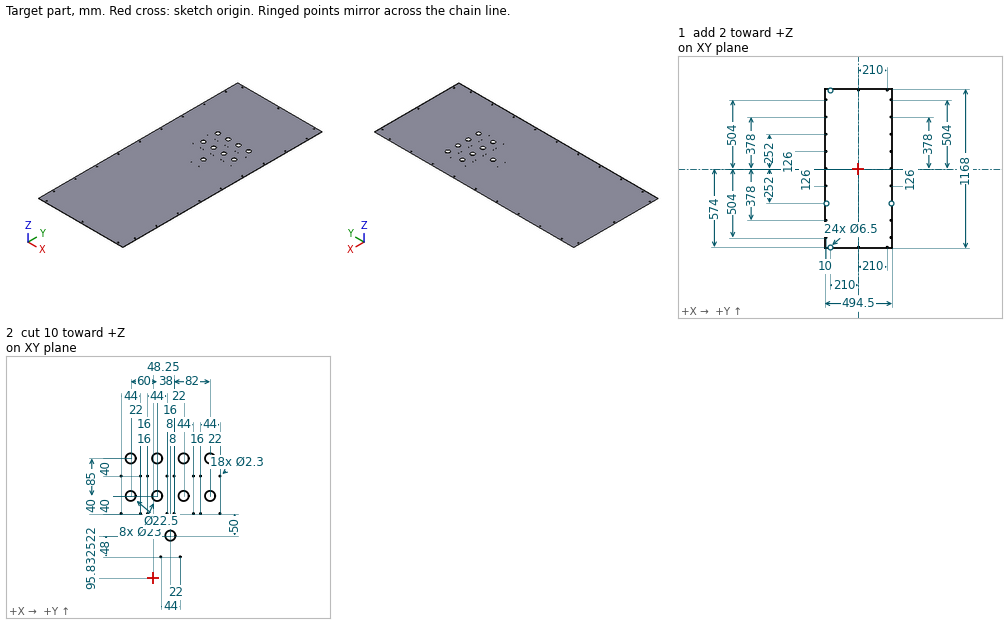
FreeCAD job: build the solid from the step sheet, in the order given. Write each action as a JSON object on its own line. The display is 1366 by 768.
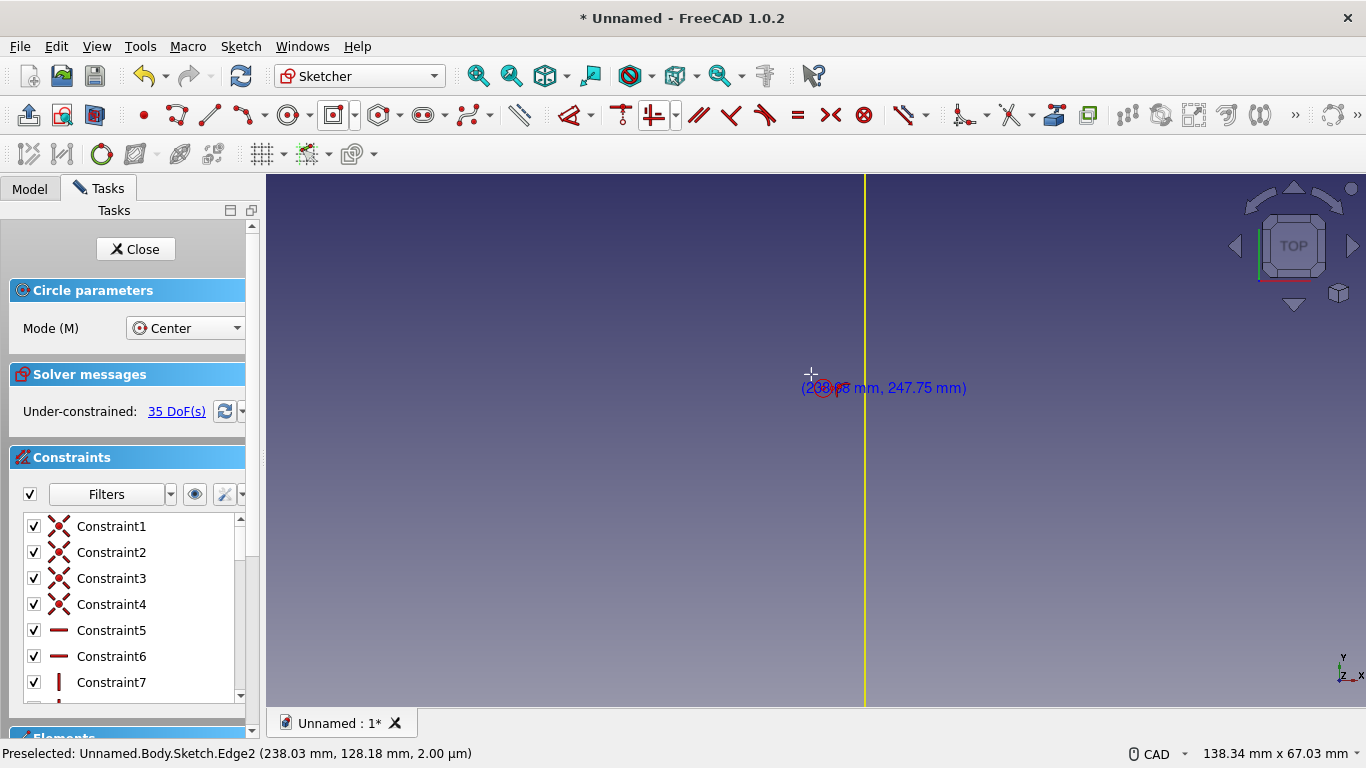
{"action": "scroll", "coordinate": [826, 359], "scroll_direction": "down", "scroll_amount": 16}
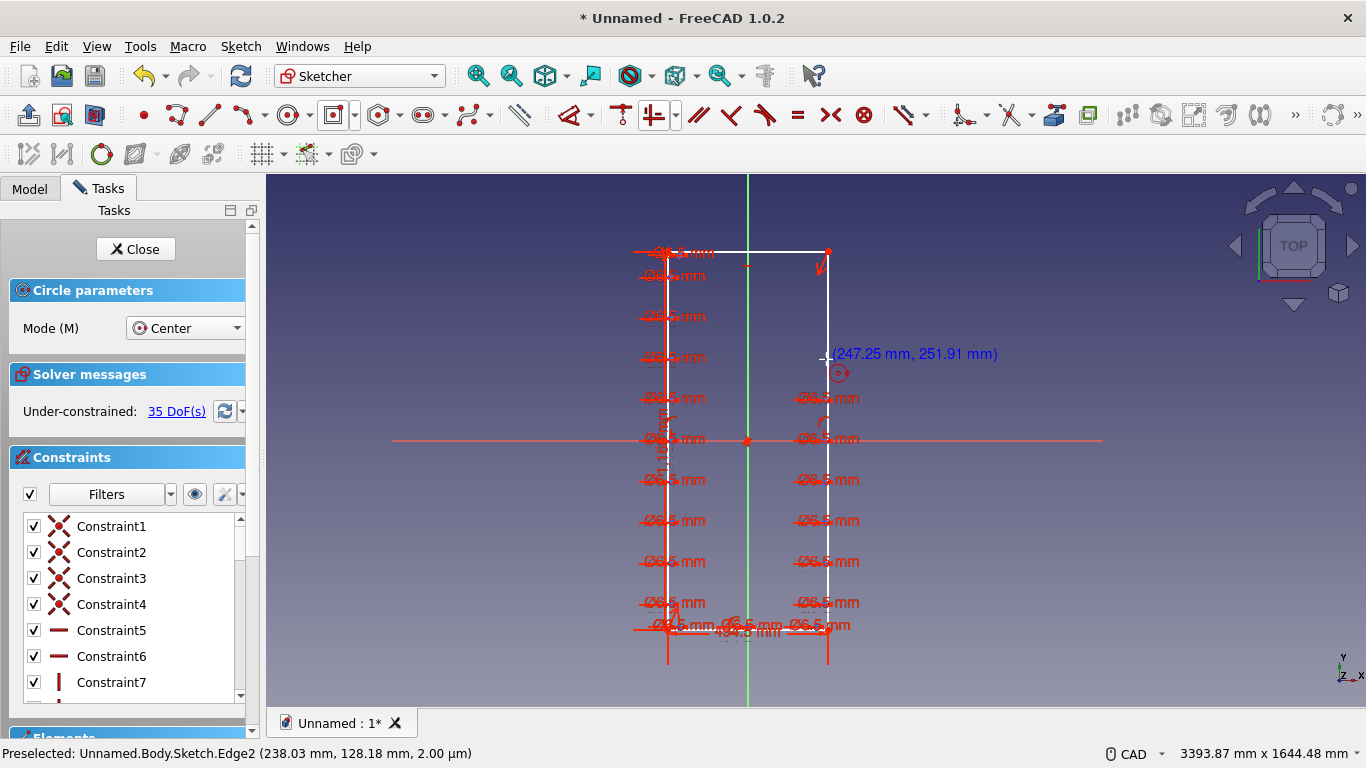
{"action": "scroll", "coordinate": [825, 359], "scroll_direction": "up", "scroll_amount": 8}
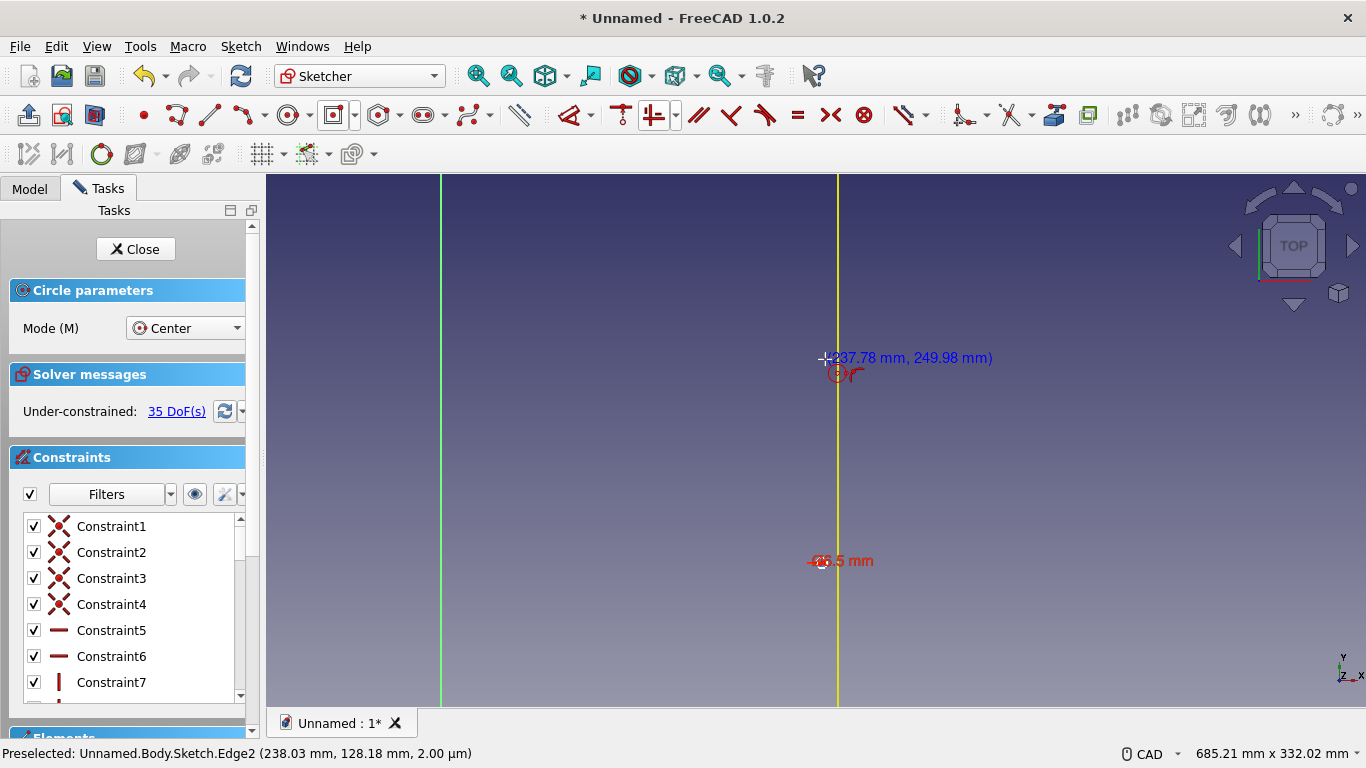
{"action": "left_click", "coordinate": [822, 359]}
{"action": "mouse_move", "coordinate": [818, 356]}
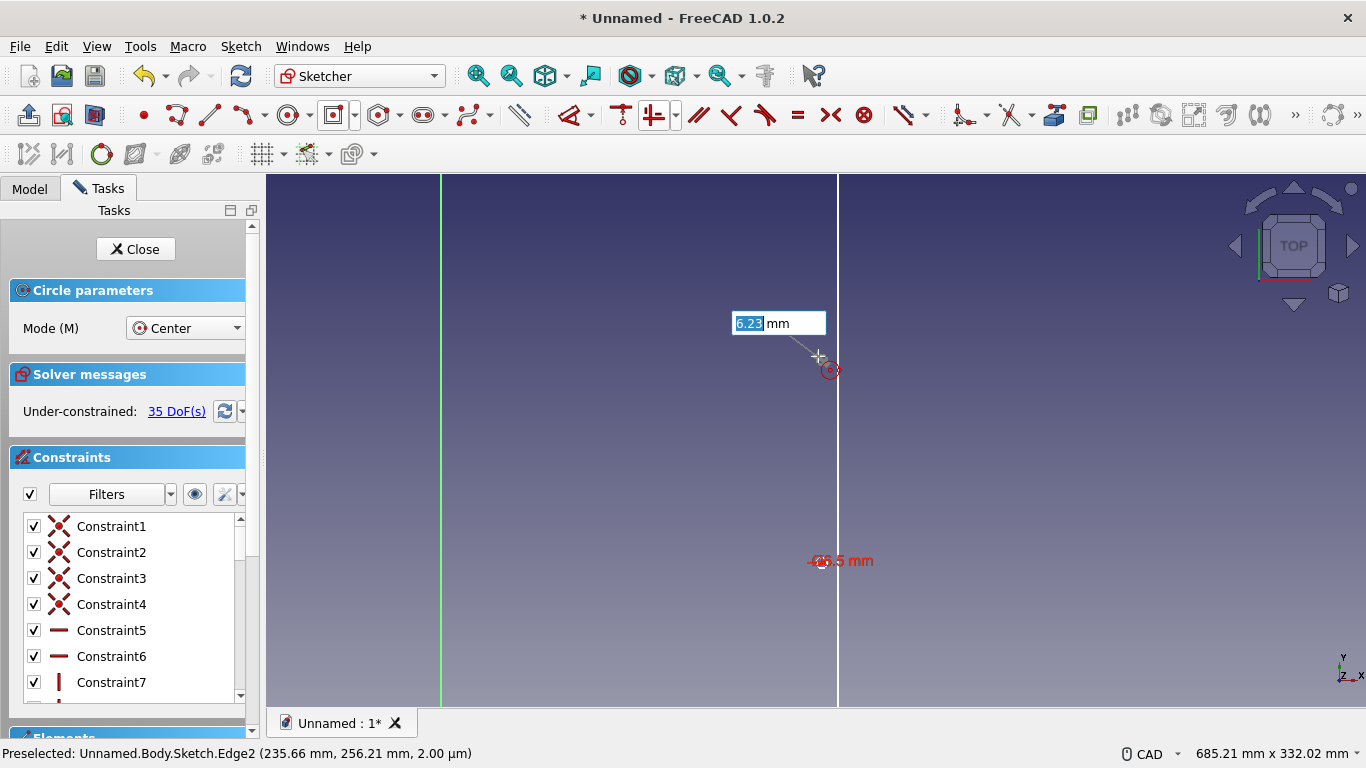
{"action": "type", "text": "6.5"}
{"action": "key", "text": "Return"}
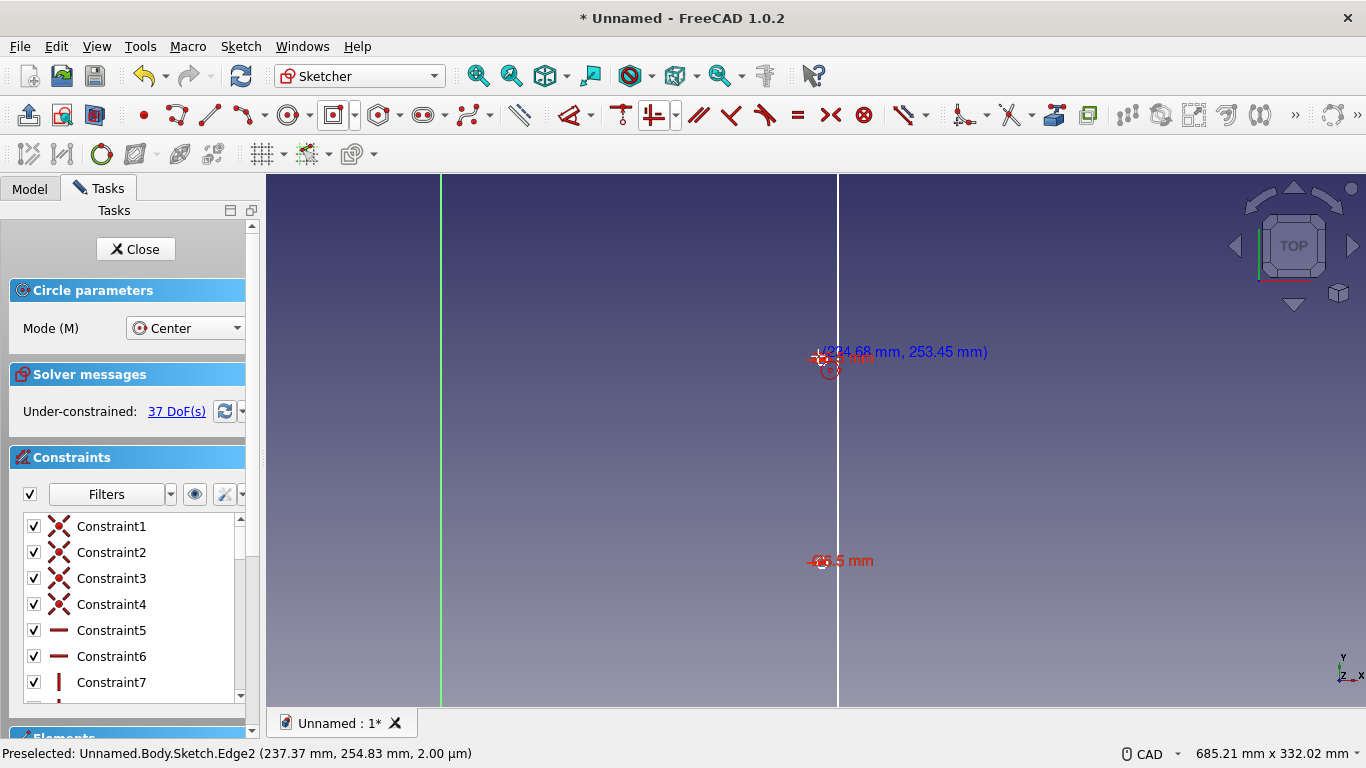
{"action": "scroll", "coordinate": [808, 376], "scroll_direction": "down", "scroll_amount": 9}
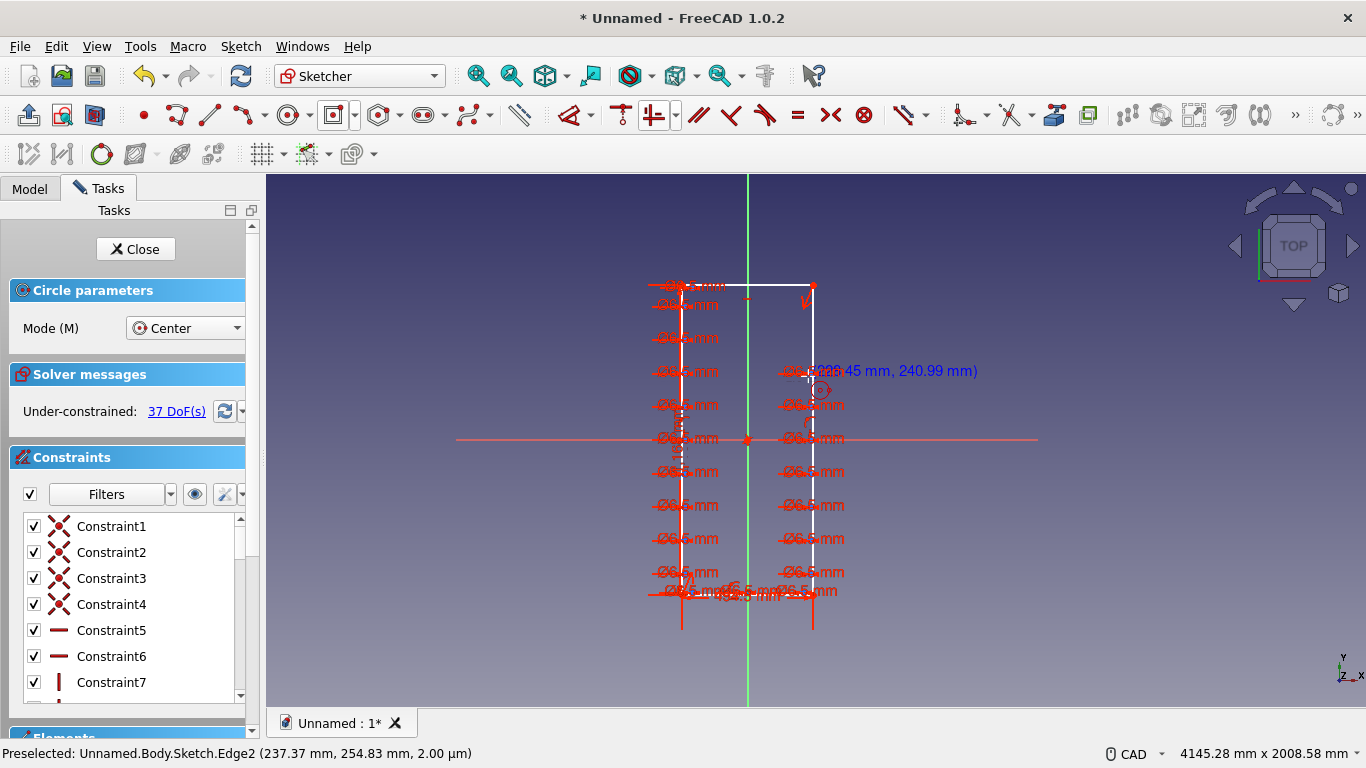
{"action": "scroll", "coordinate": [748, 288], "scroll_direction": "up", "scroll_amount": 17}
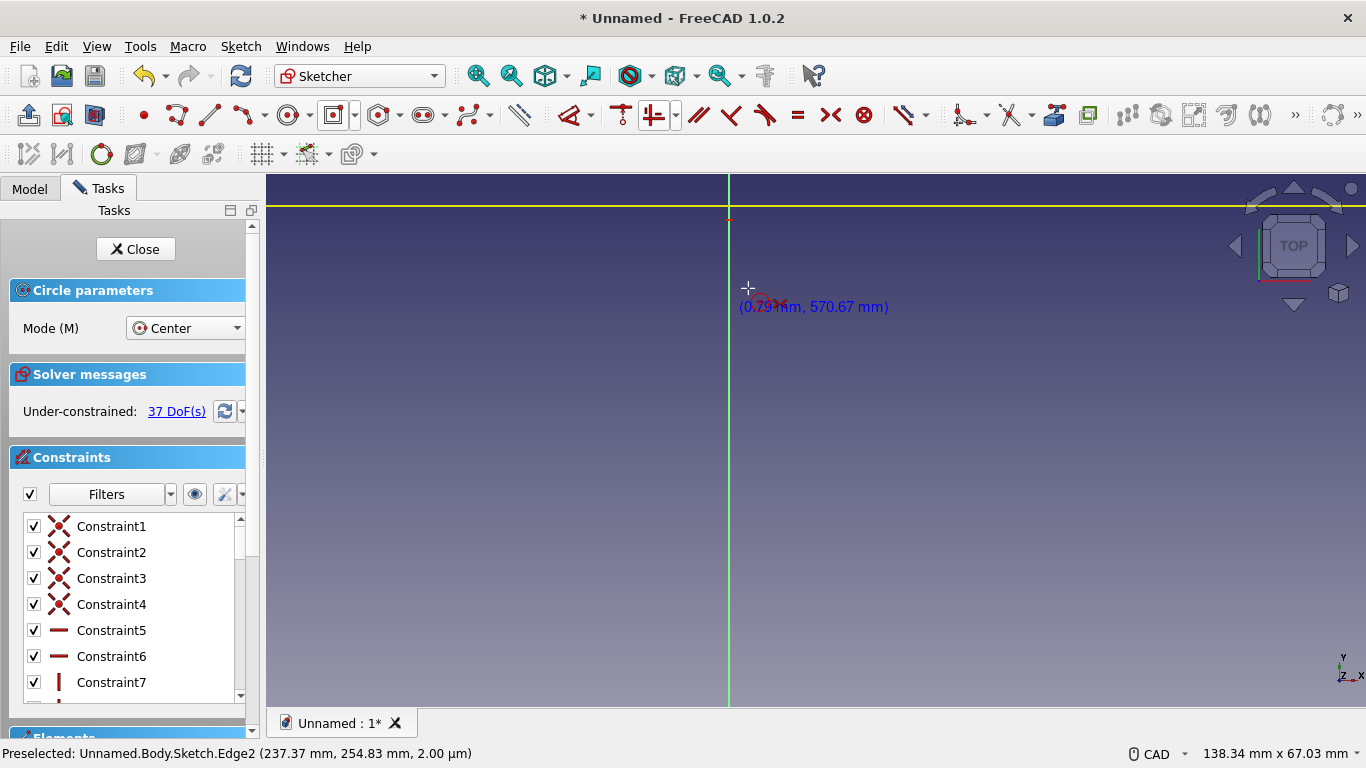
{"action": "scroll", "coordinate": [748, 253], "scroll_direction": "down", "scroll_amount": 16}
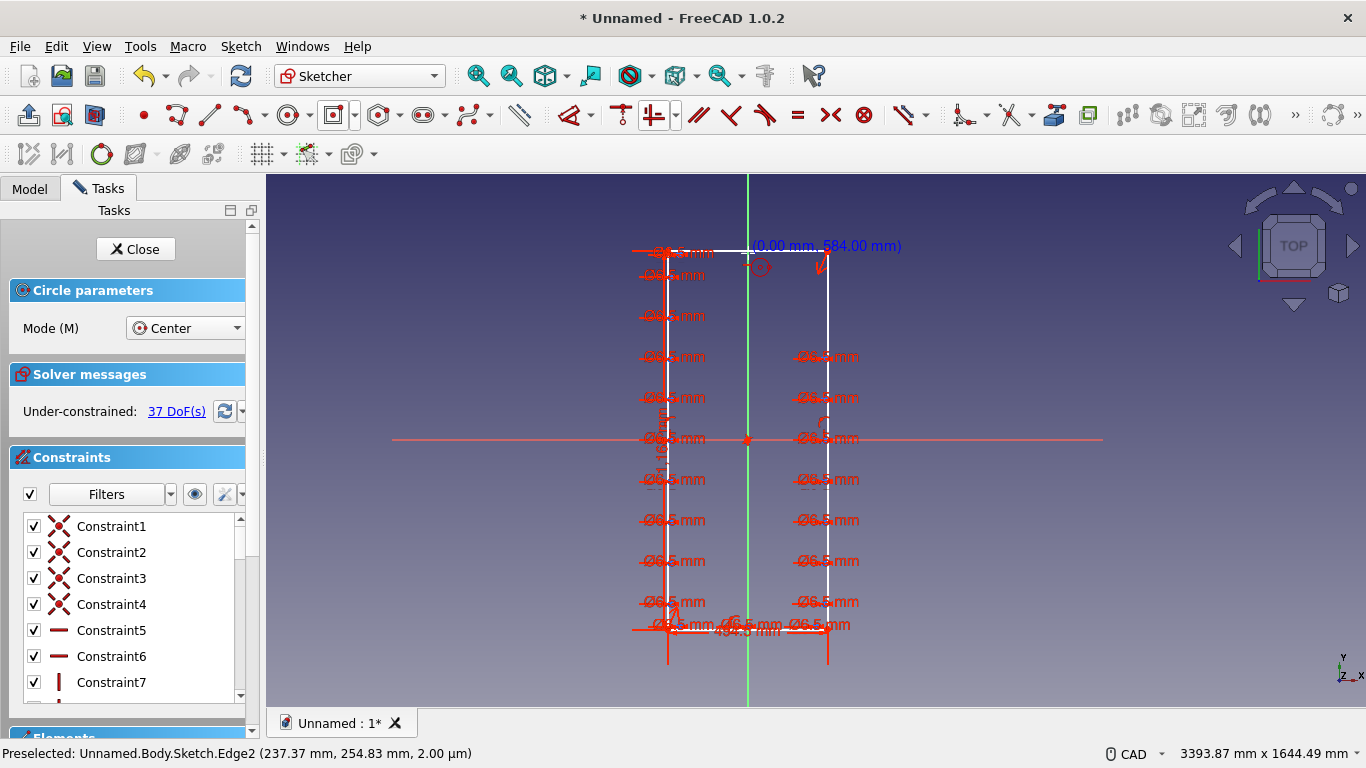
{"action": "scroll", "coordinate": [748, 254], "scroll_direction": "up", "scroll_amount": 8}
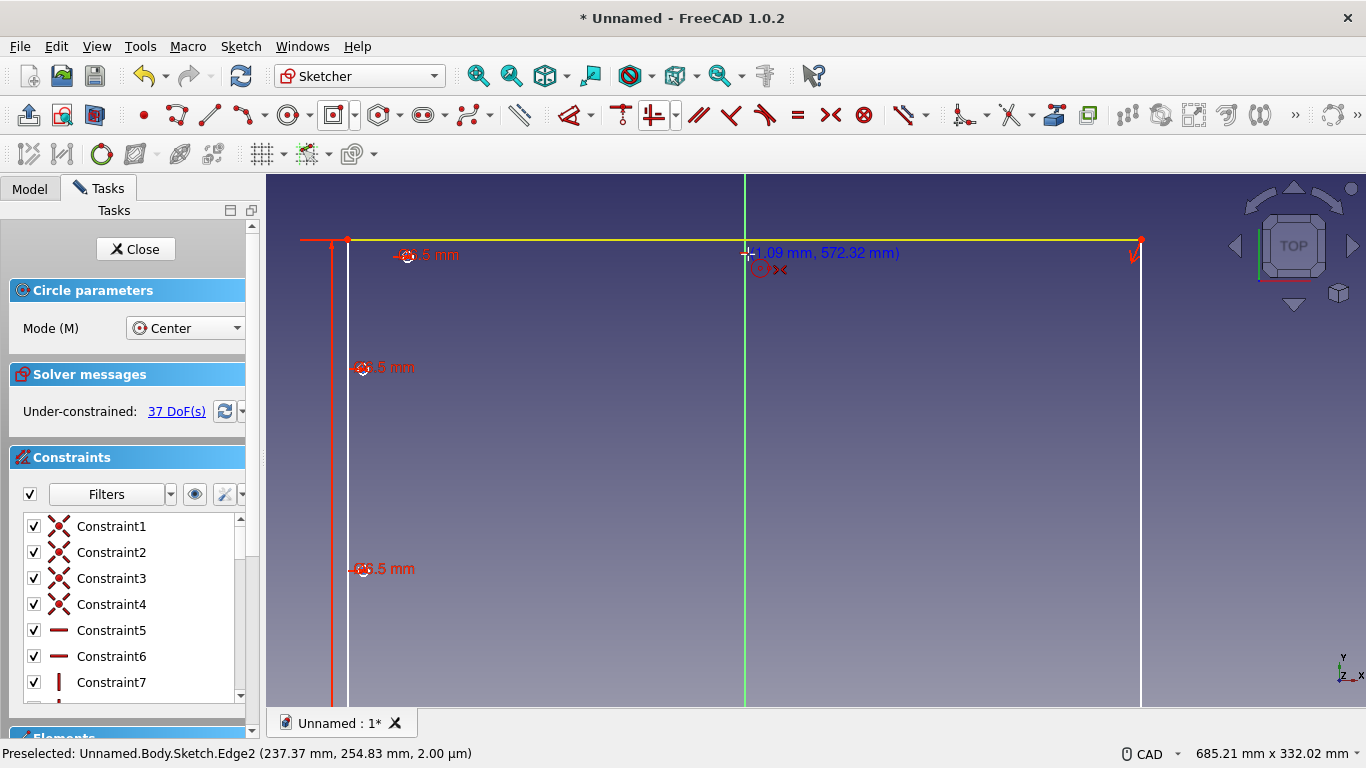
{"action": "left_click", "coordinate": [745, 256]}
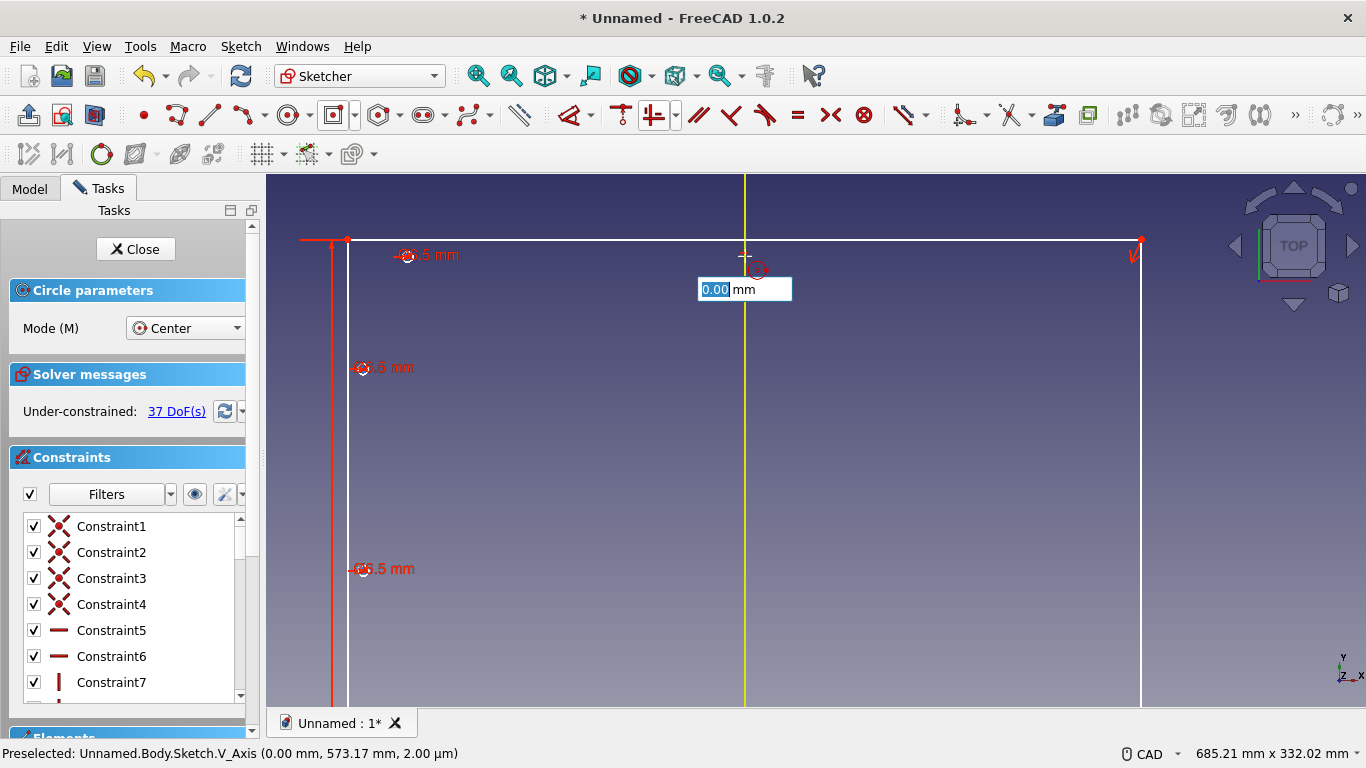
{"action": "scroll", "coordinate": [749, 254], "scroll_direction": "up", "scroll_amount": 6}
{"action": "mouse_move", "coordinate": [749, 253]}